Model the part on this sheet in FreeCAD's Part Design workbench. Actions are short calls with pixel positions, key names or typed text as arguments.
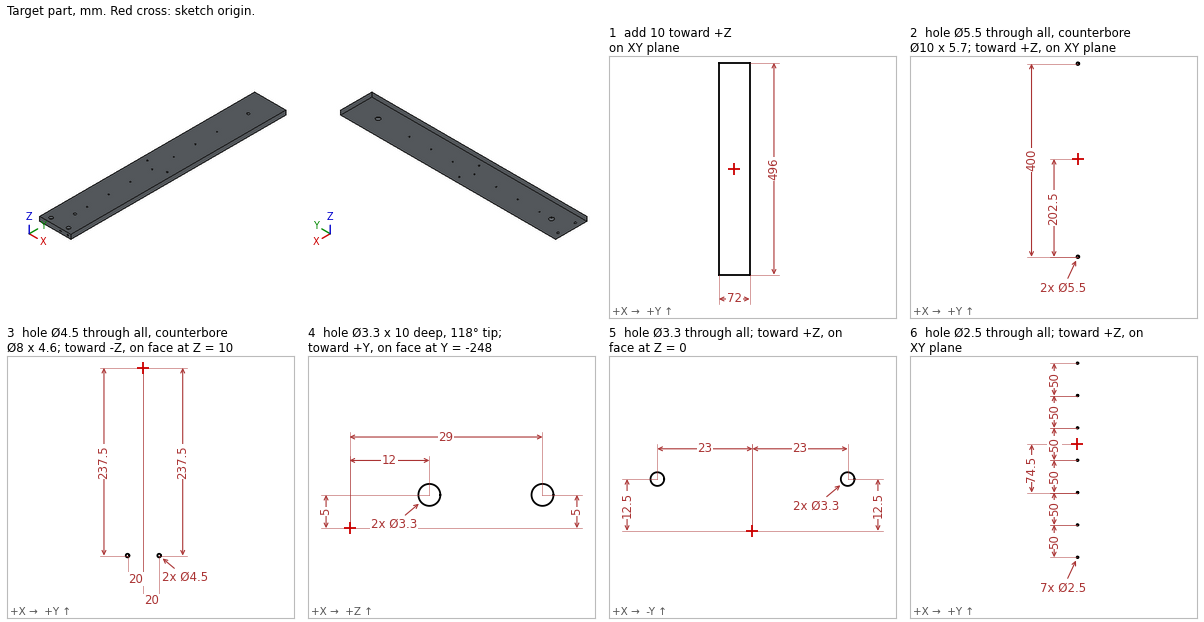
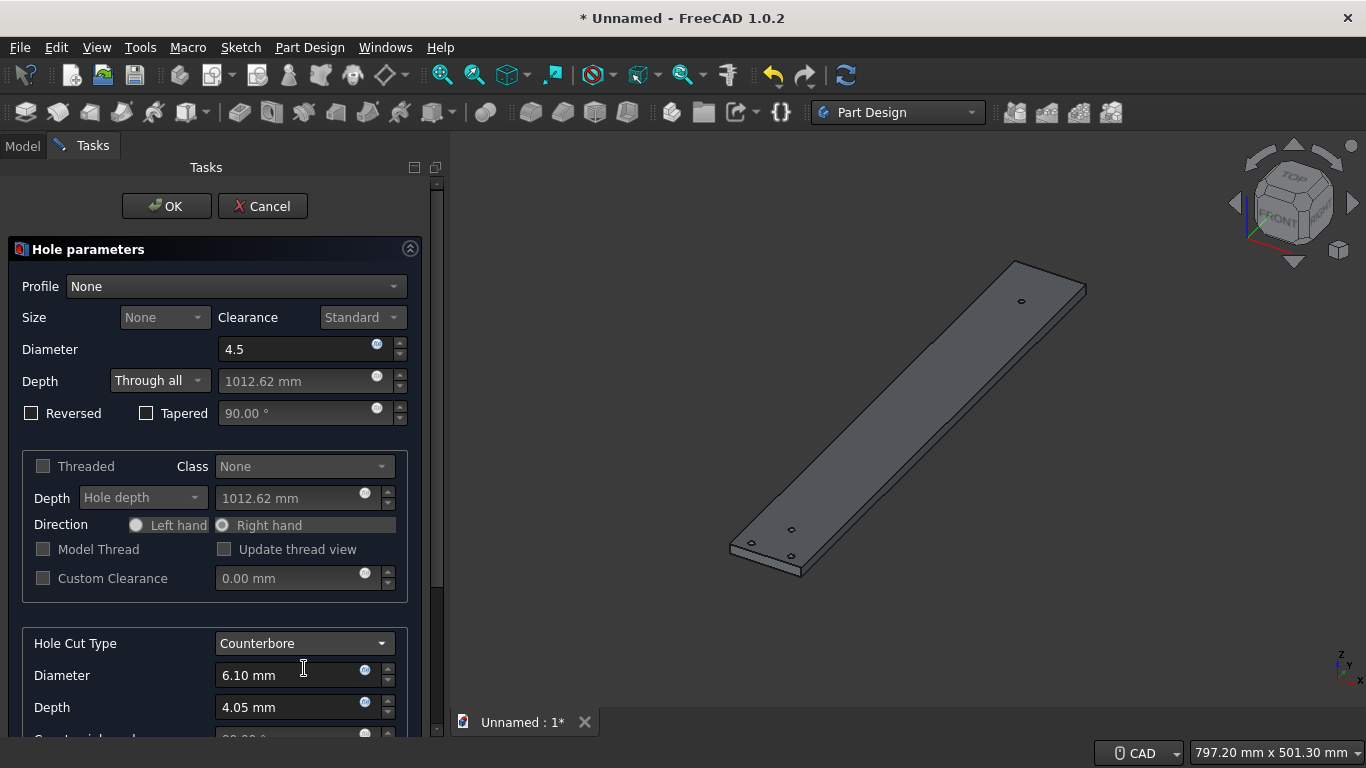
triple_click(298, 675)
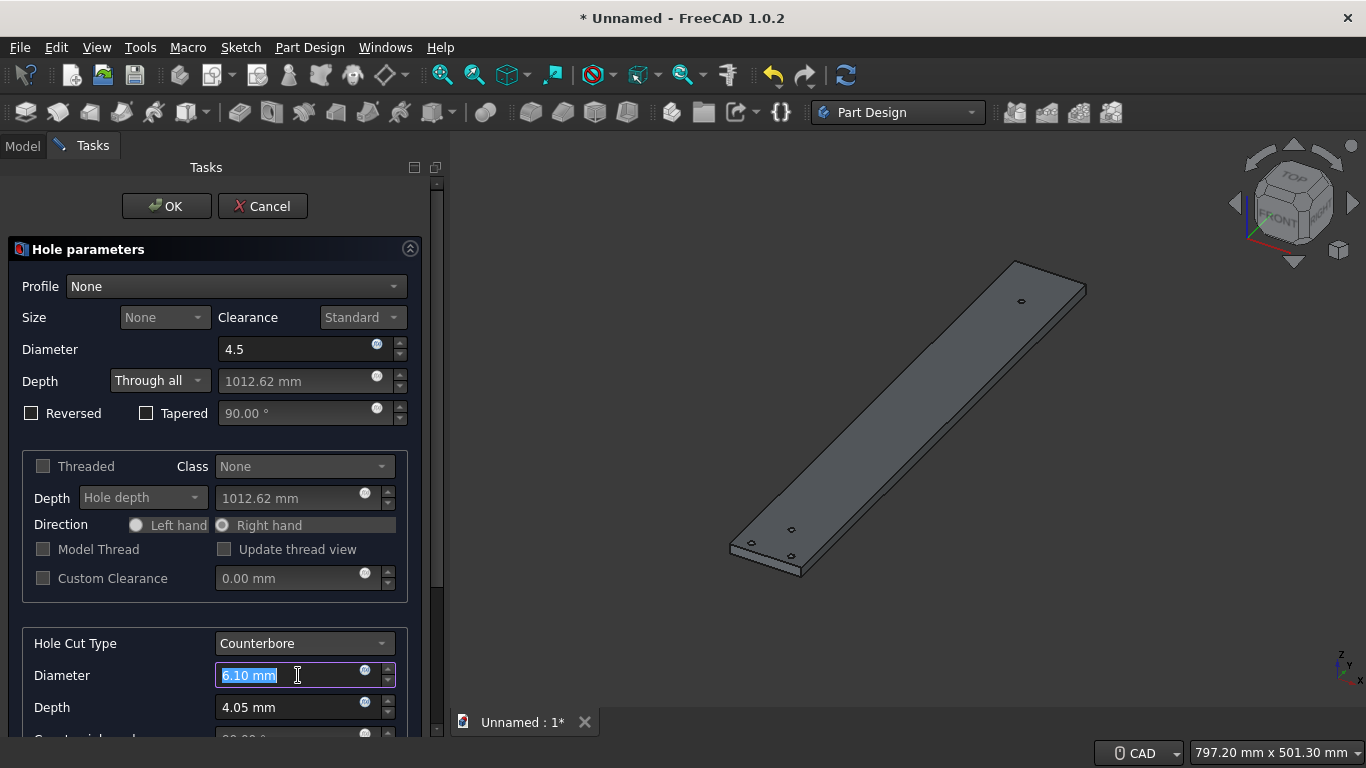
text(8)
key(Tab)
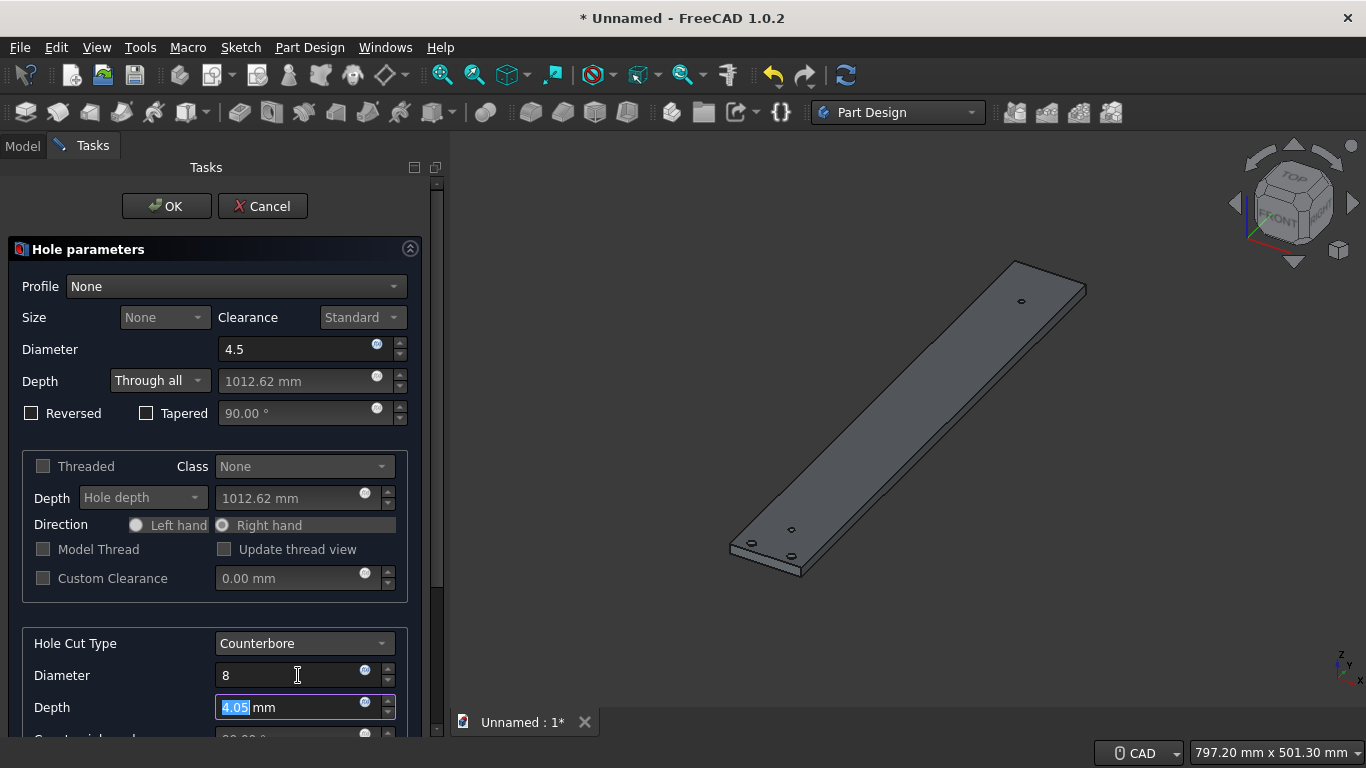
text(4.6)
key(Tab)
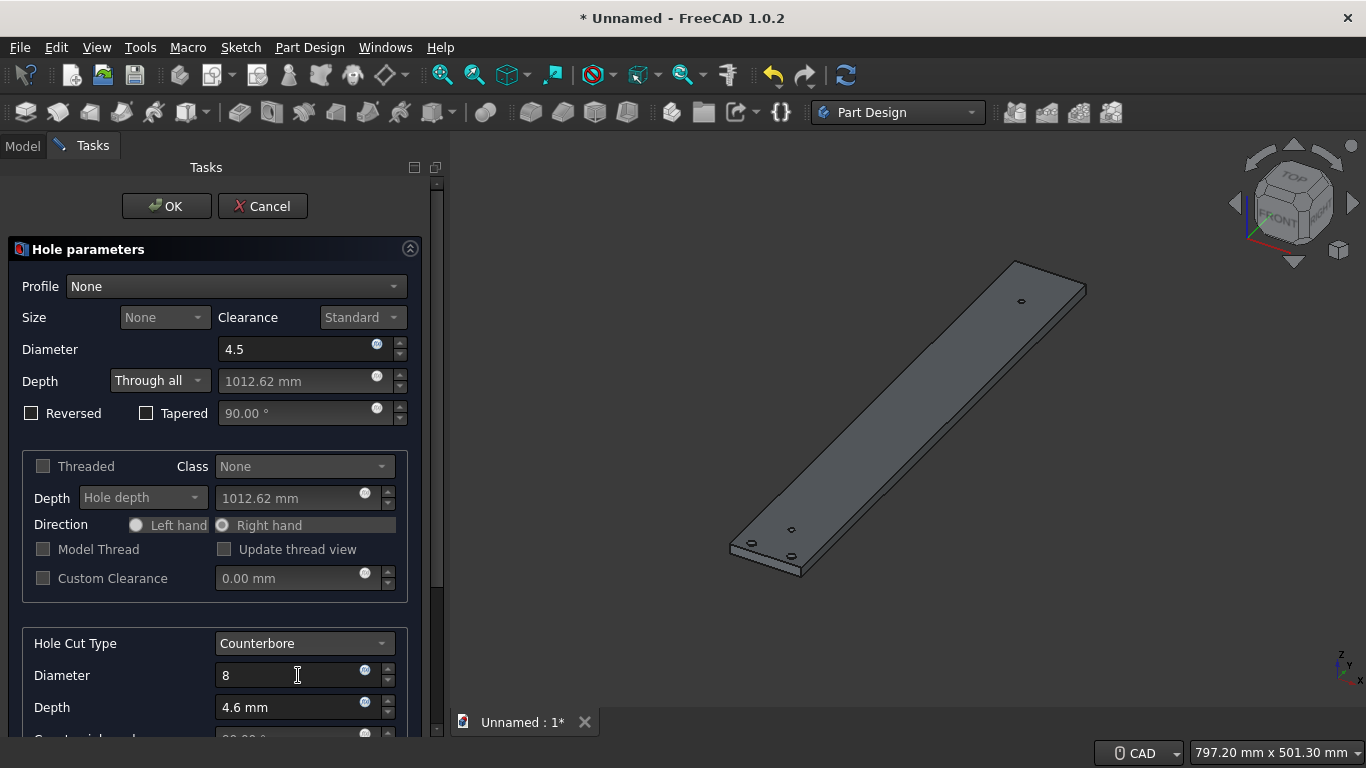
click(167, 206)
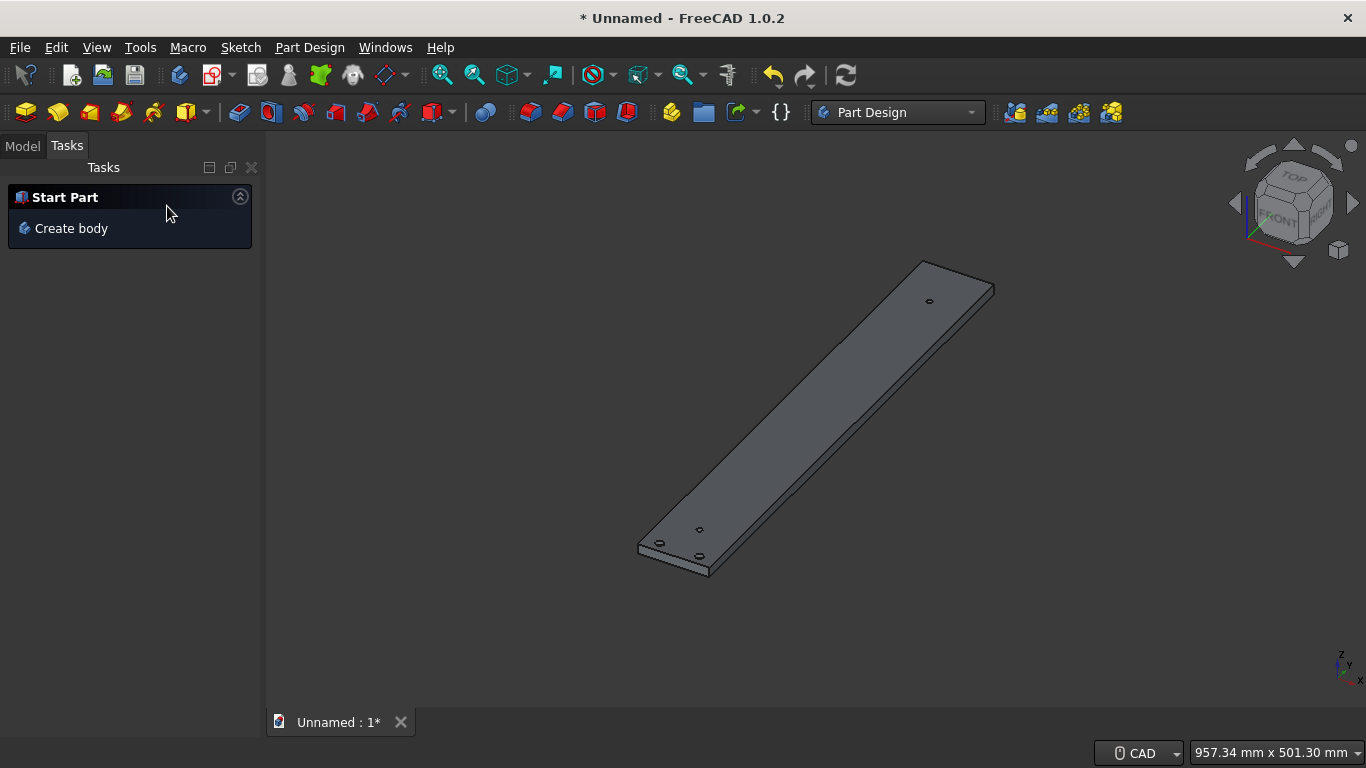
scroll(704, 570, up, 4)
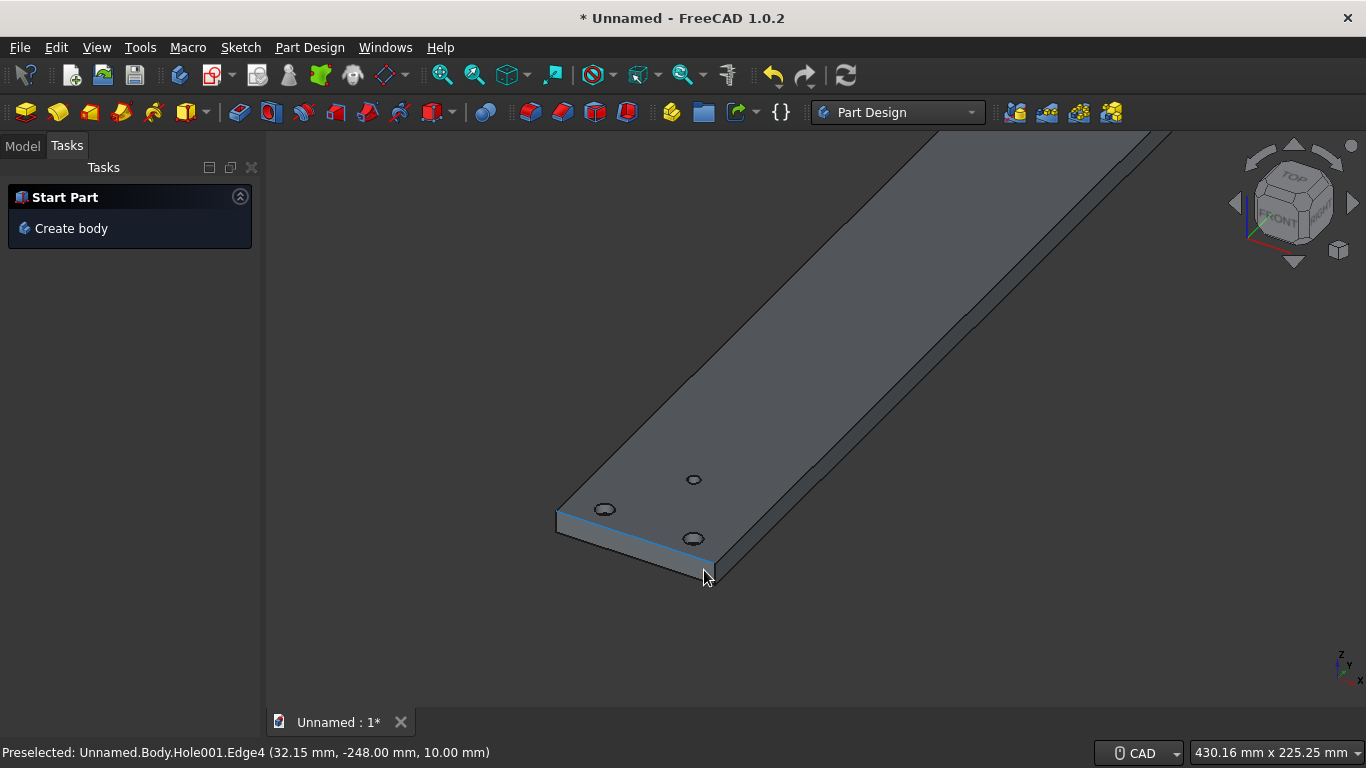
click(704, 570)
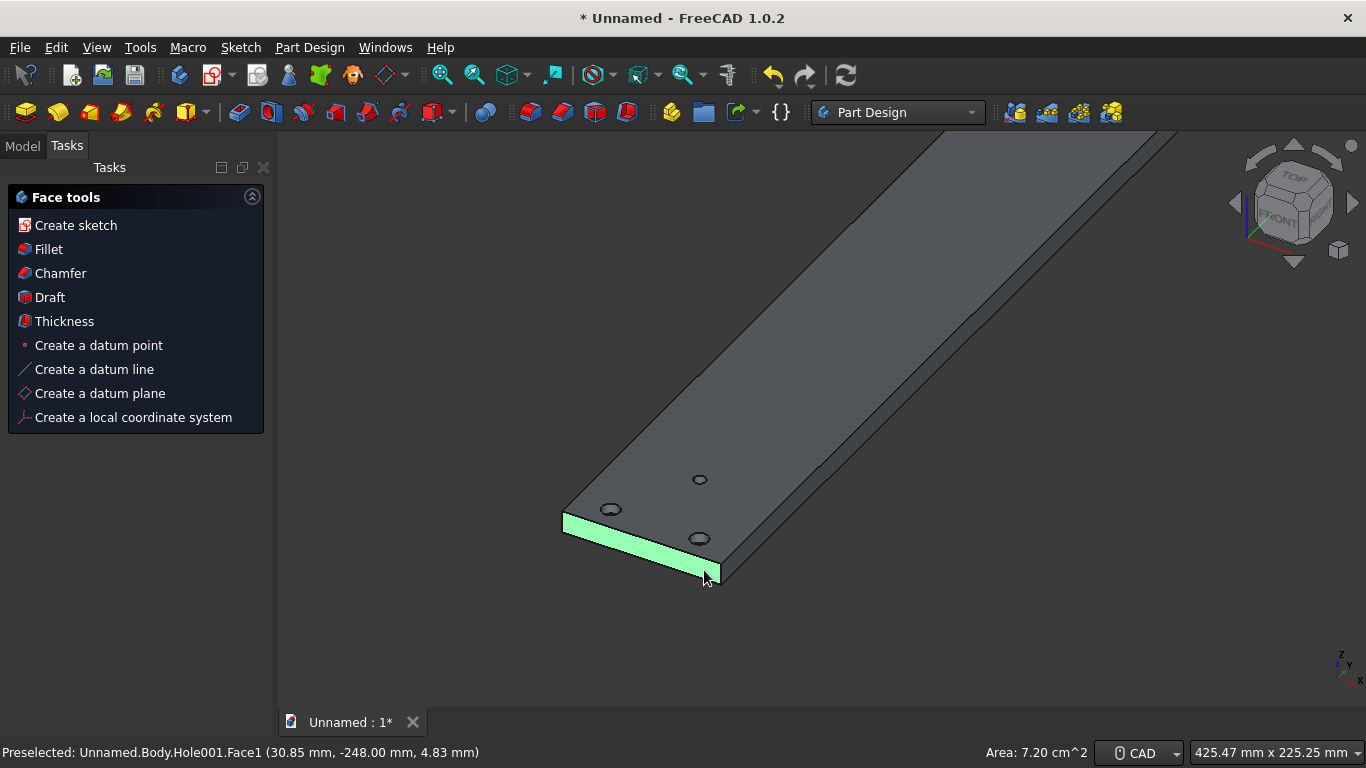
click(212, 76)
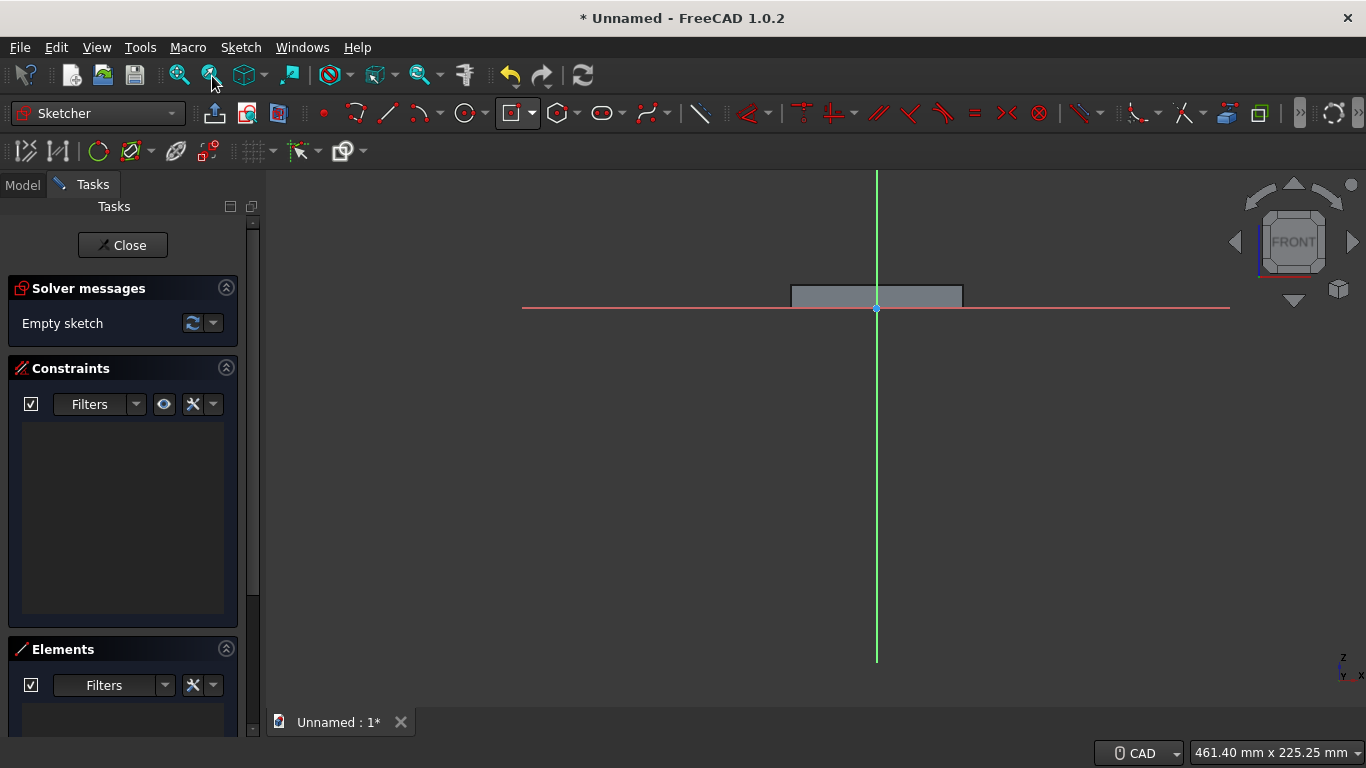
scroll(934, 283, up, 11)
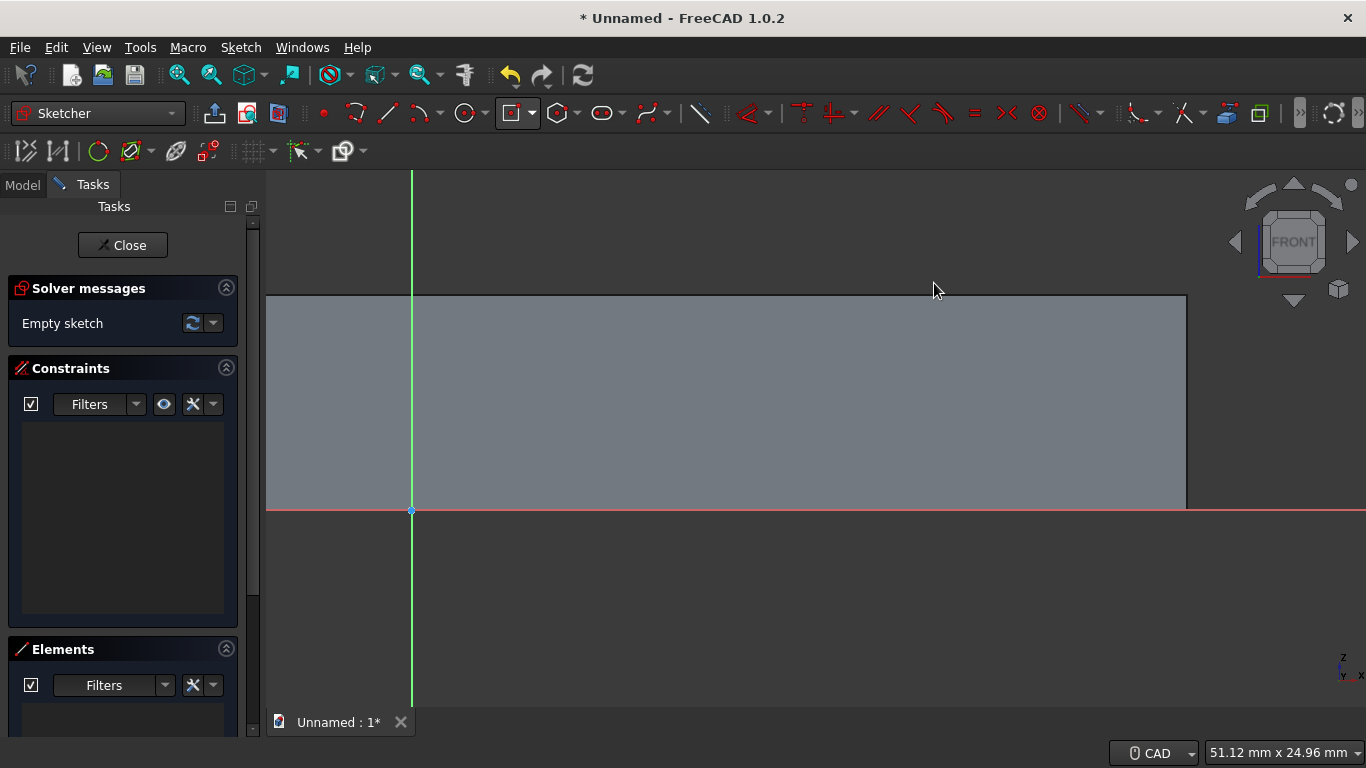
click(466, 114)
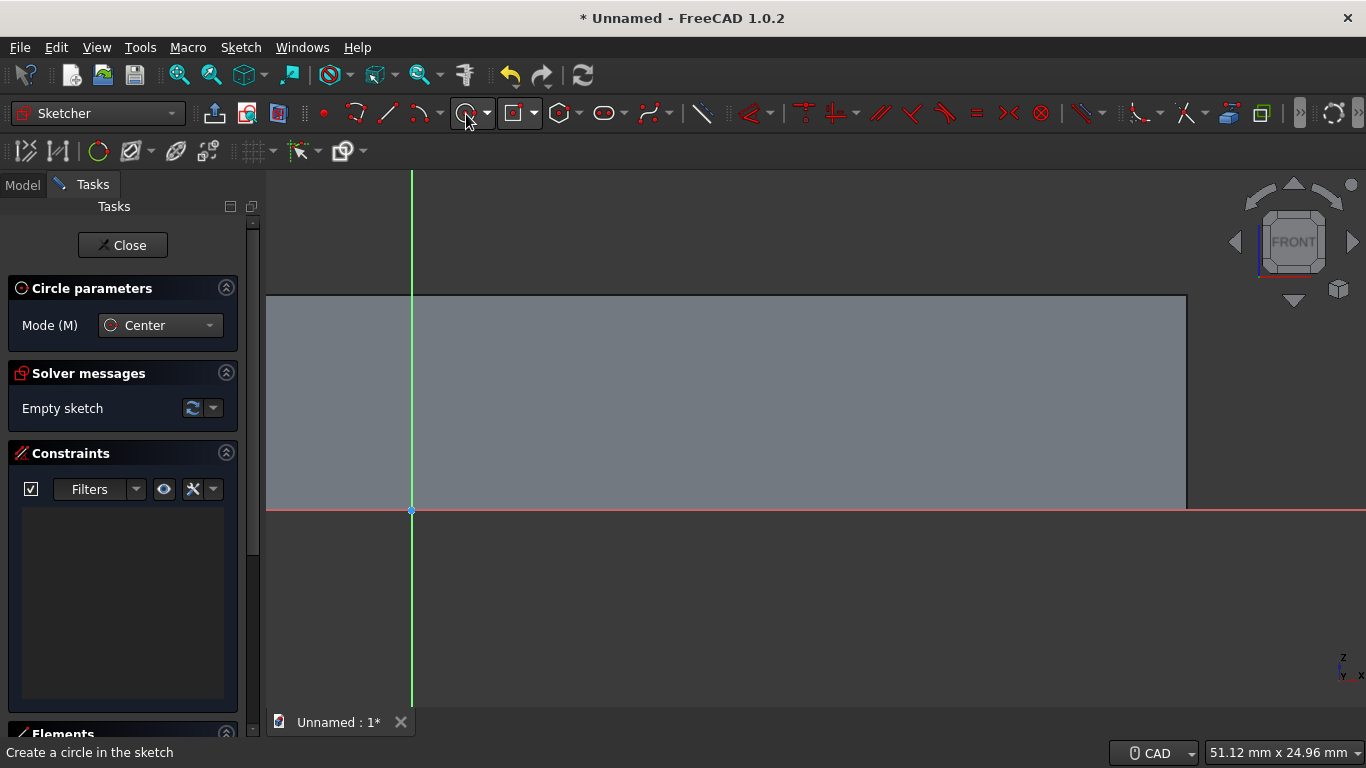
click(670, 403)
click(695, 378)